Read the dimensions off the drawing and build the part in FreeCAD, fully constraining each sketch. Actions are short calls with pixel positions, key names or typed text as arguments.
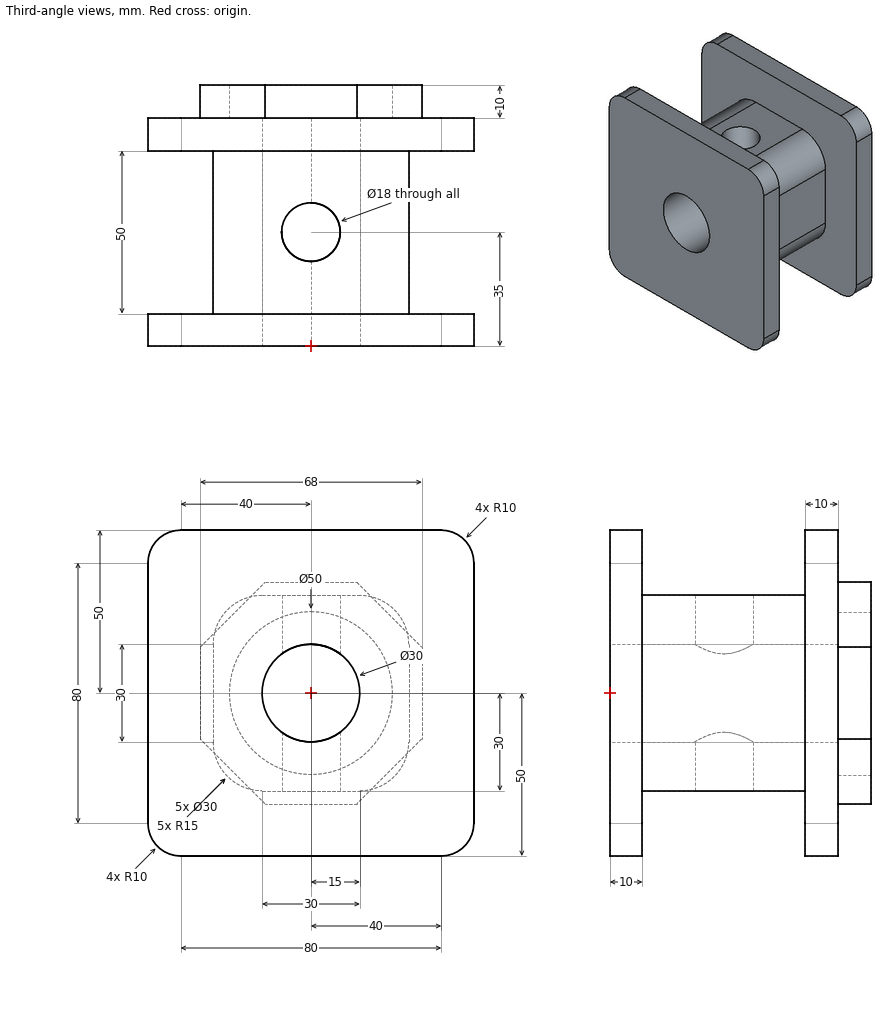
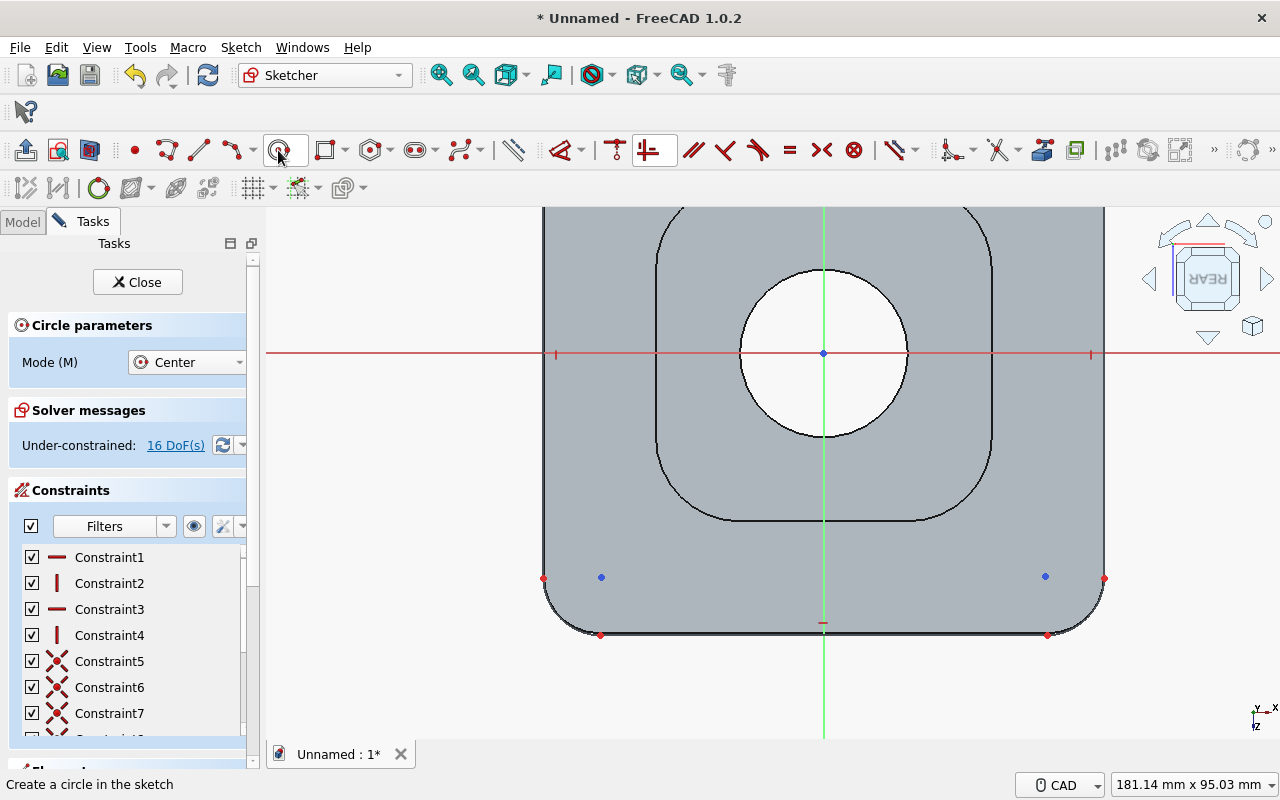
click(824, 353)
move(883, 294)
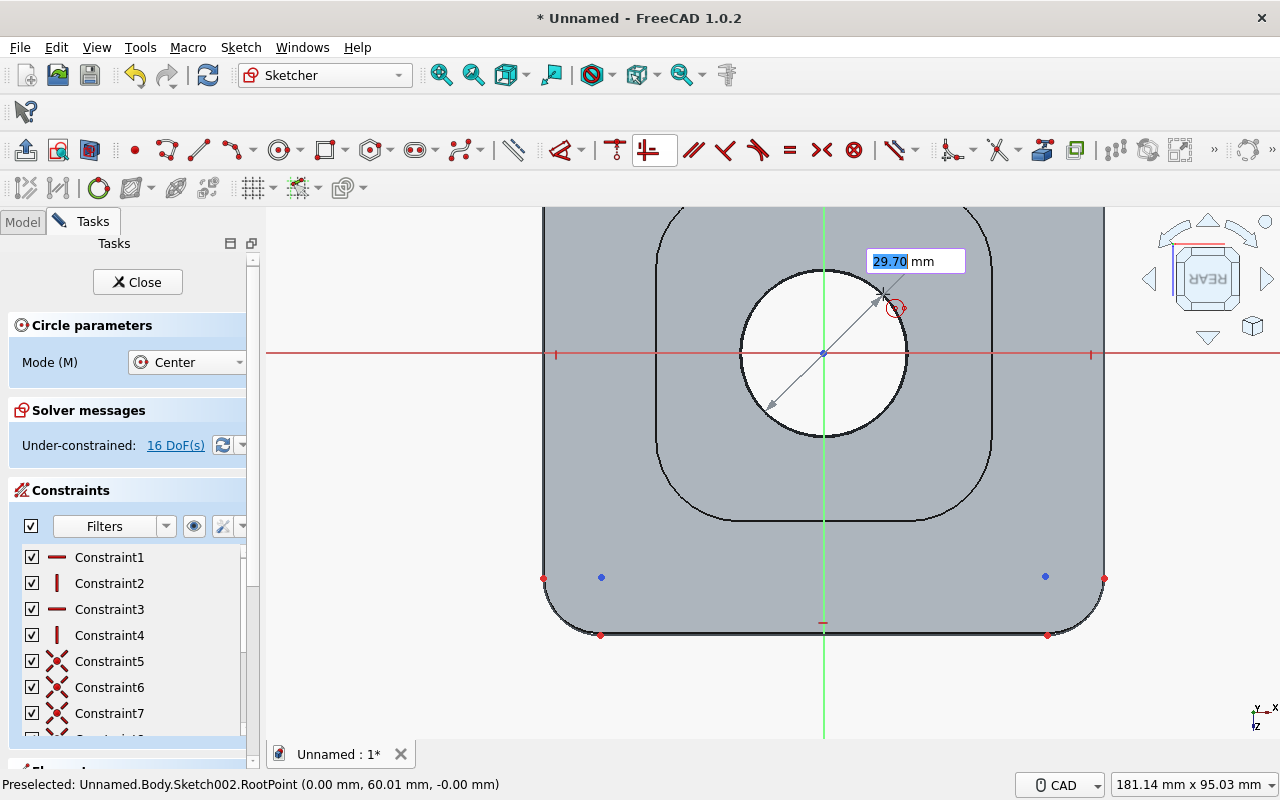
text(30)
key(Return)
key(Escape)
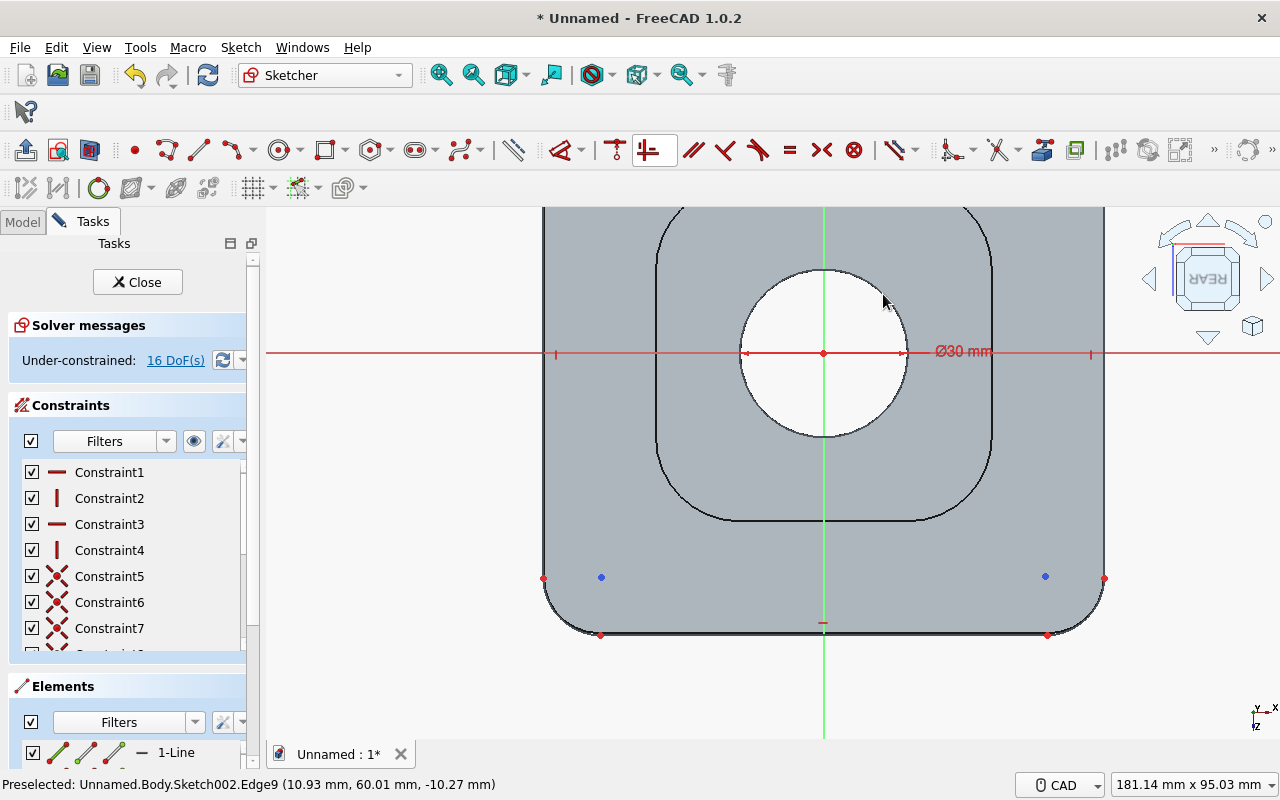
click(734, 635)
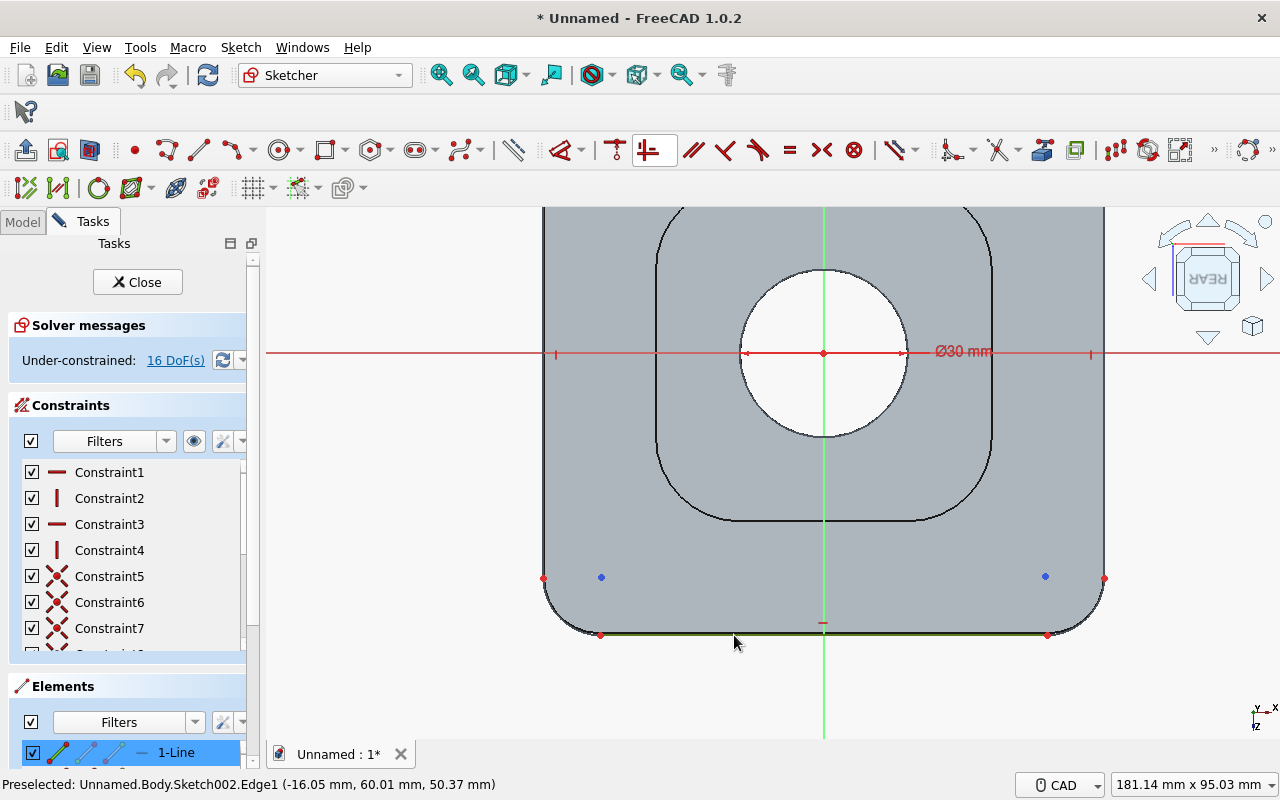
click(1073, 629)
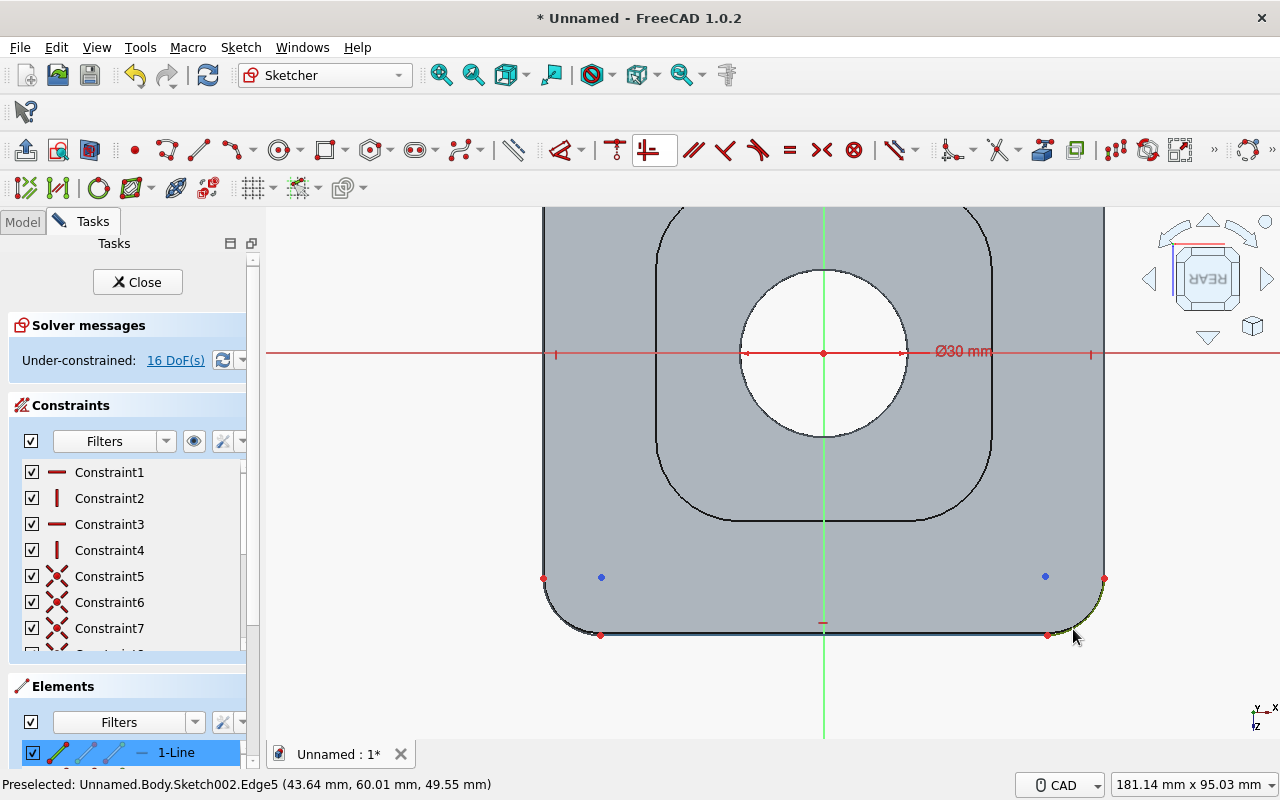
click(758, 150)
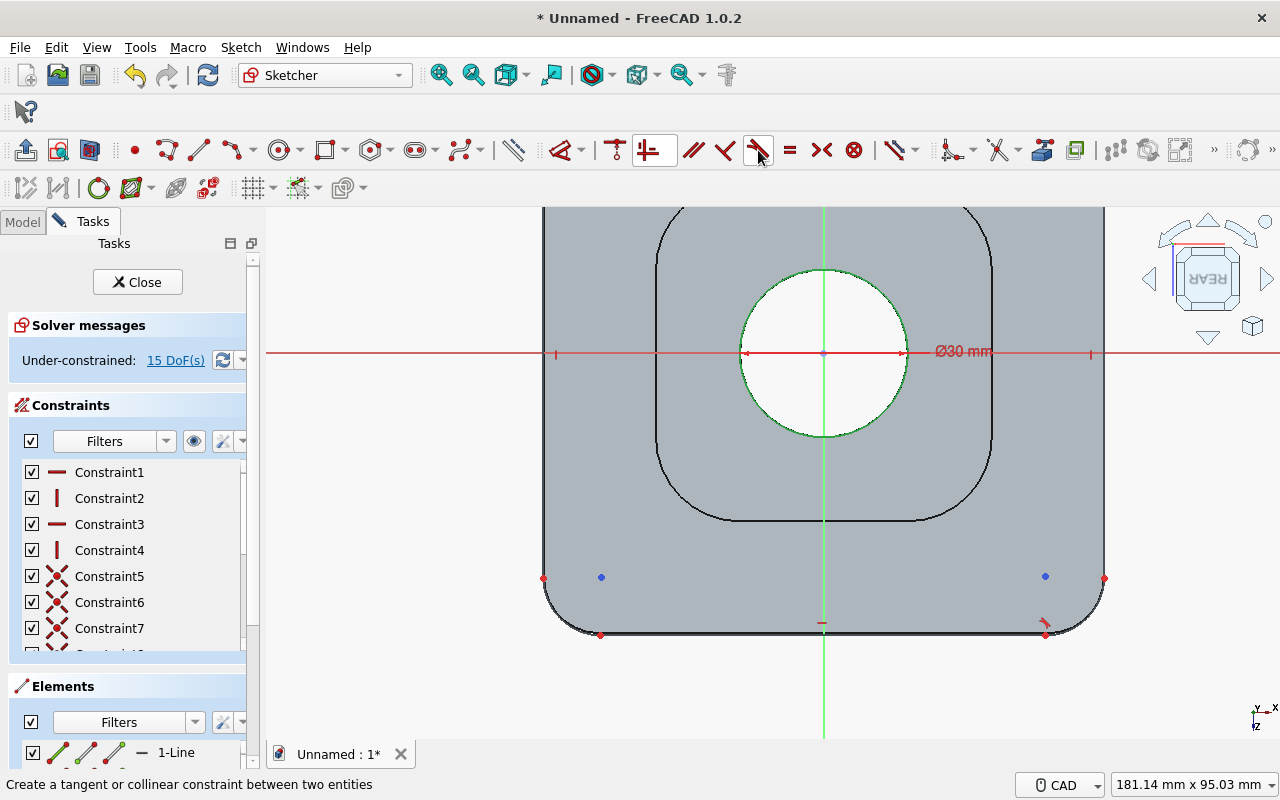
click(734, 635)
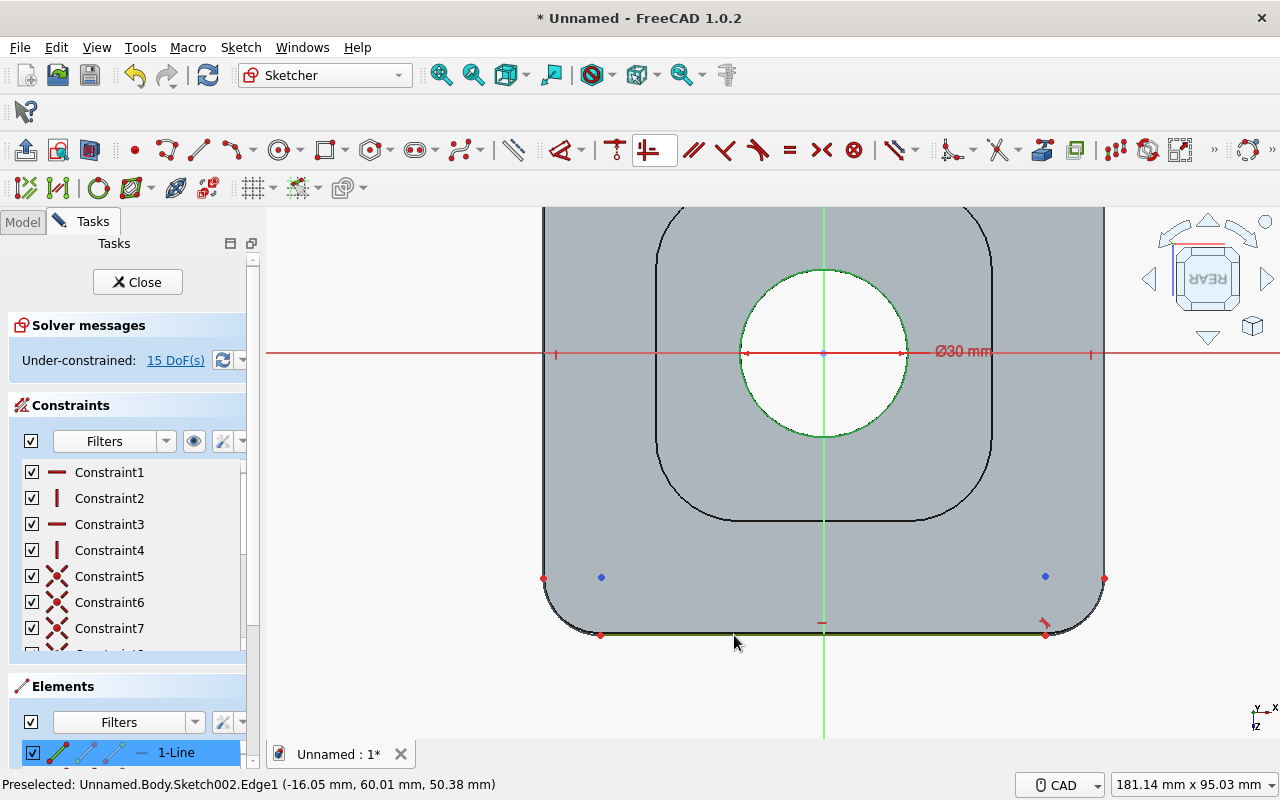
click(550, 604)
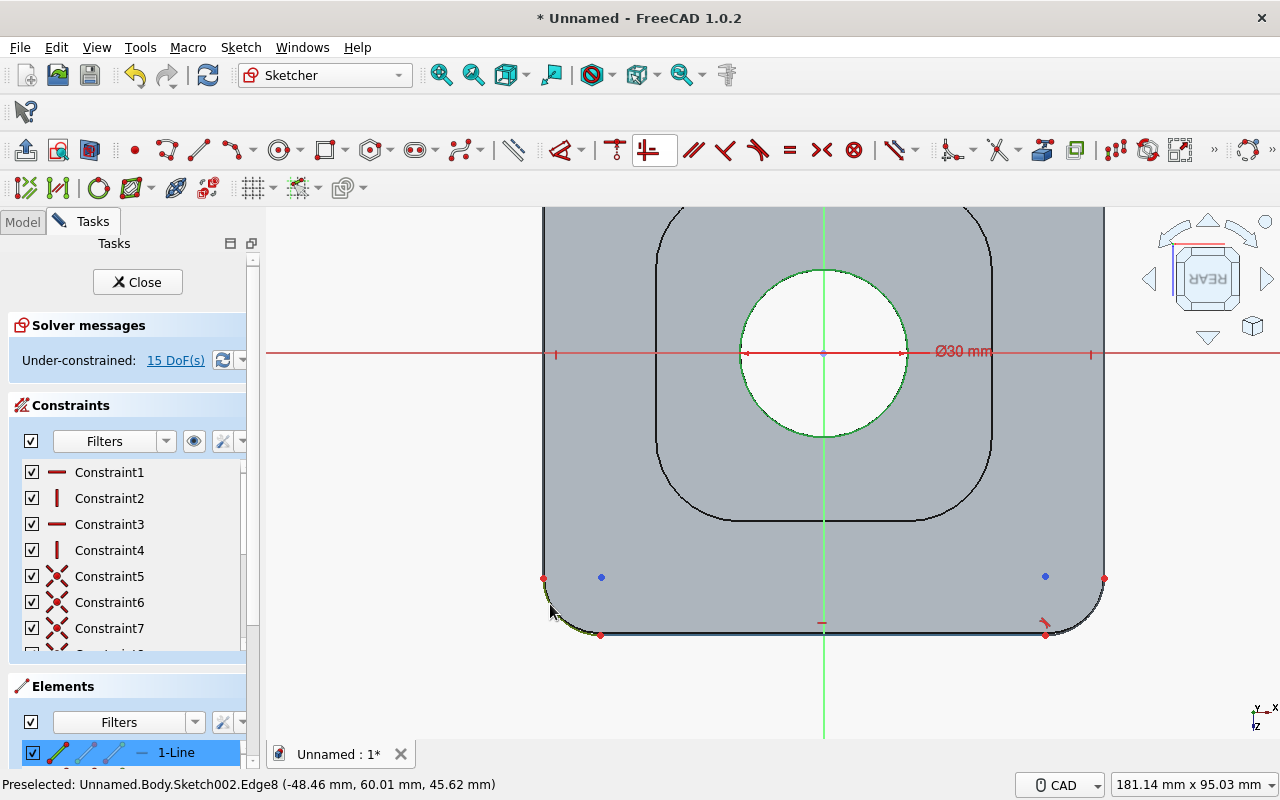
click(758, 150)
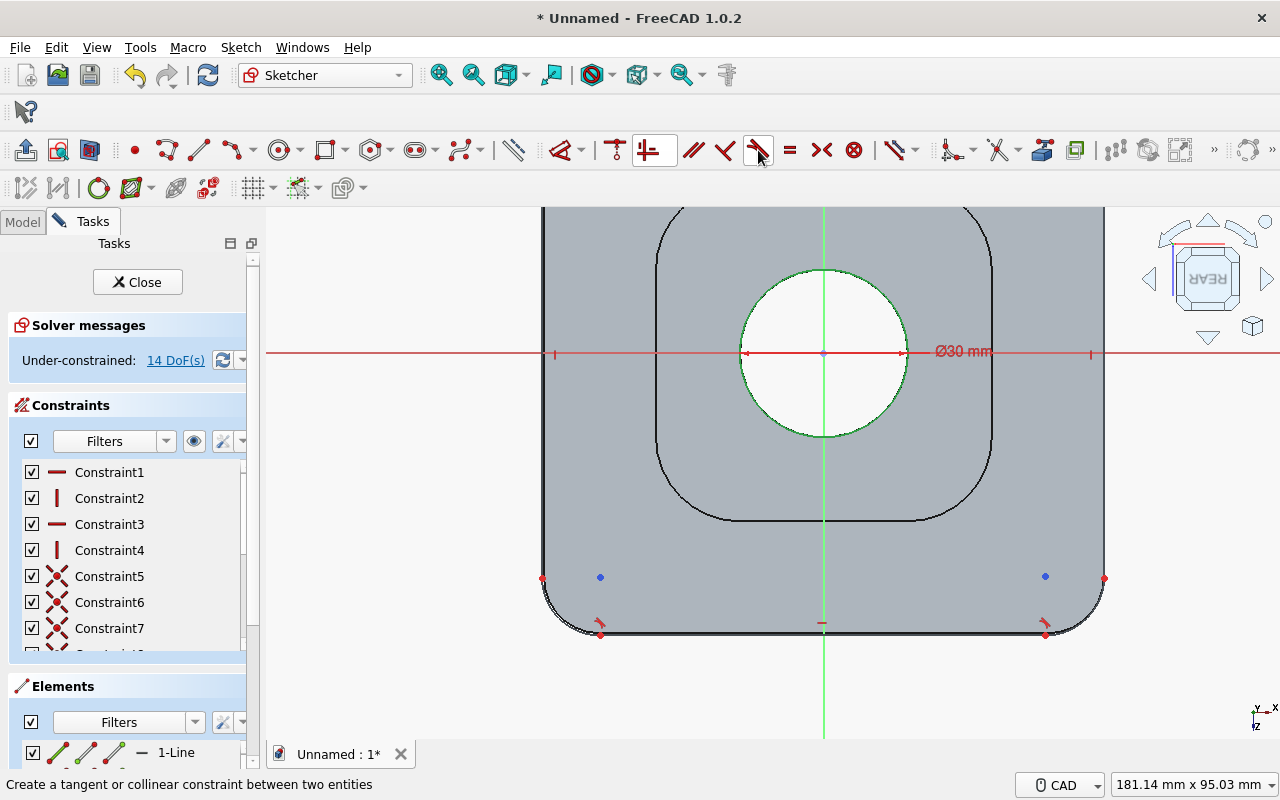
click(1104, 444)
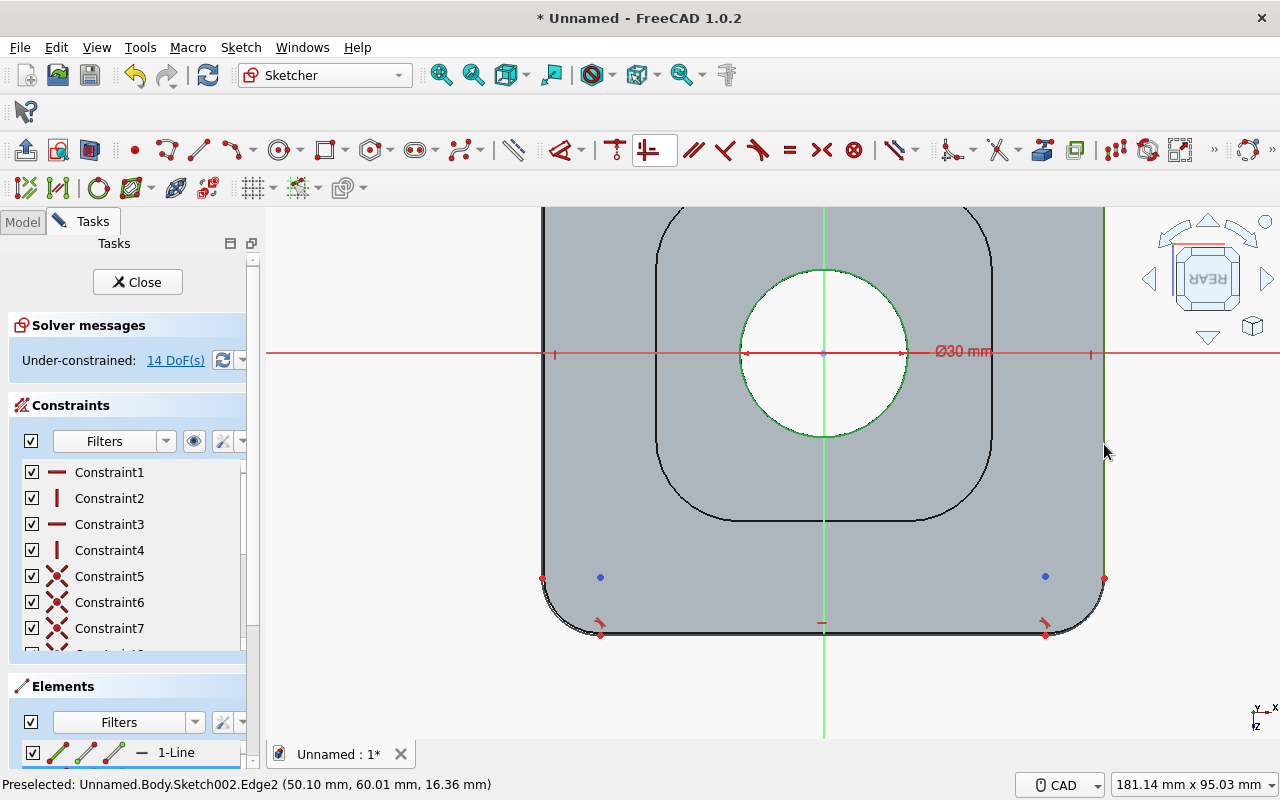
click(1071, 629)